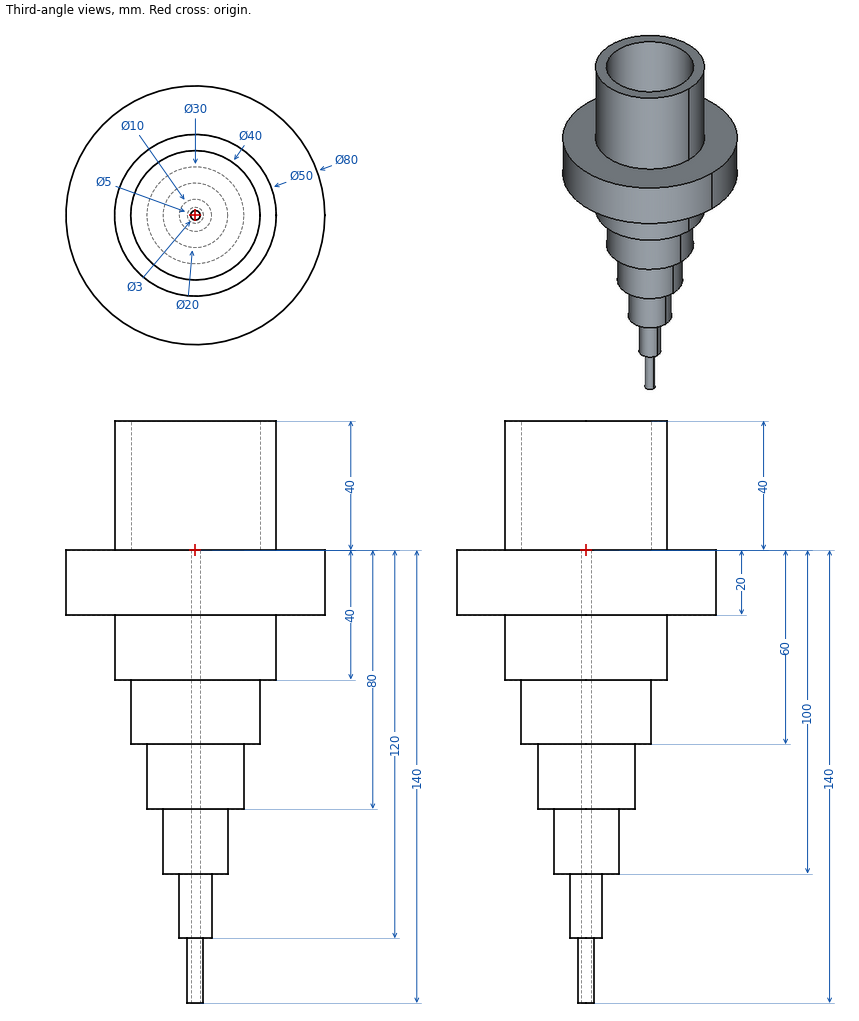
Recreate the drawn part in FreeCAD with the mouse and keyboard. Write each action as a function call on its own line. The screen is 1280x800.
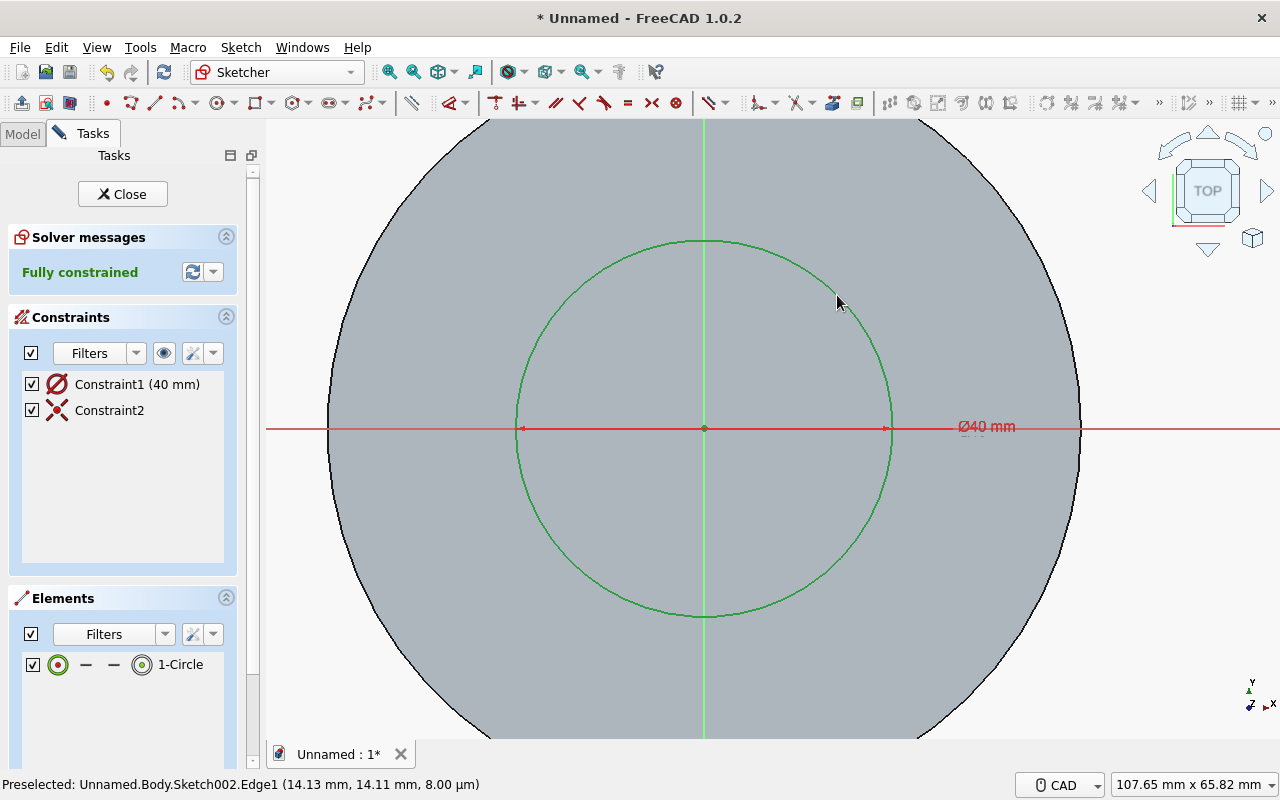
click(123, 194)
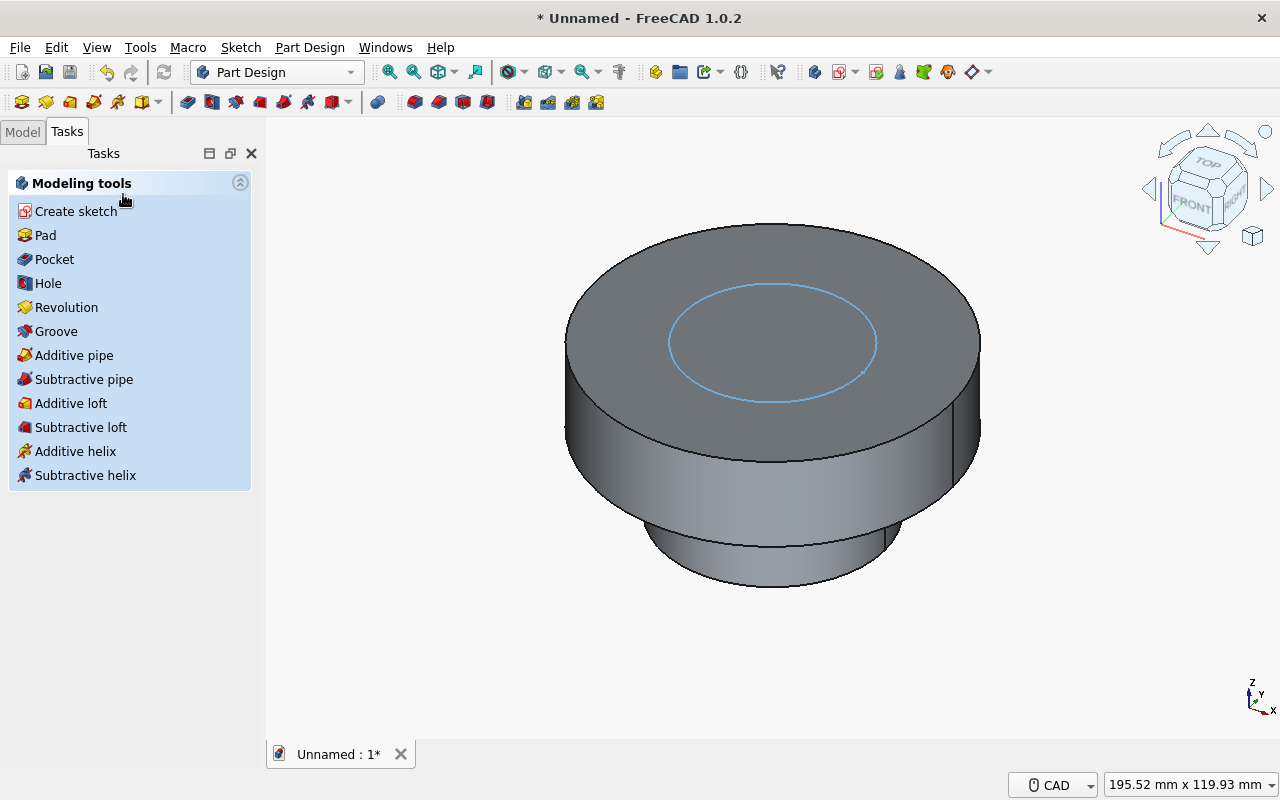
click(22, 102)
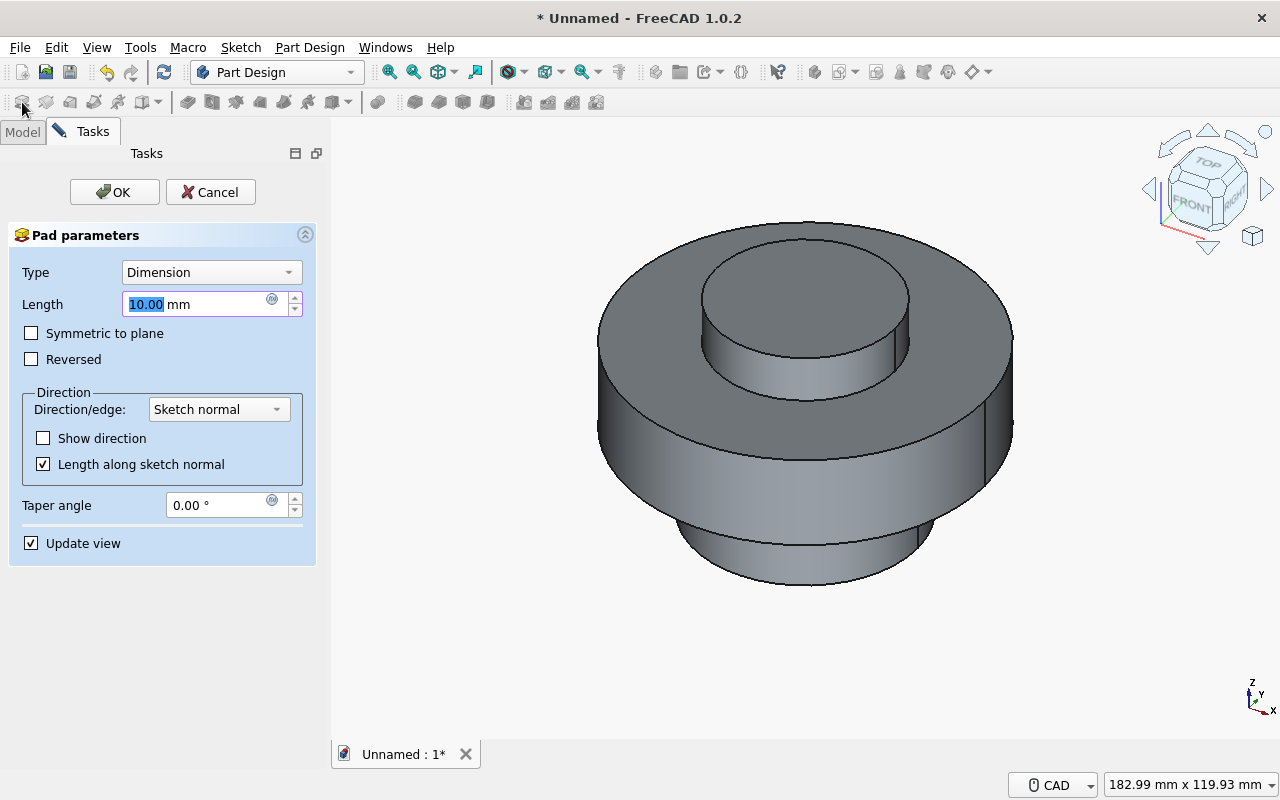
text(60)
key(Tab)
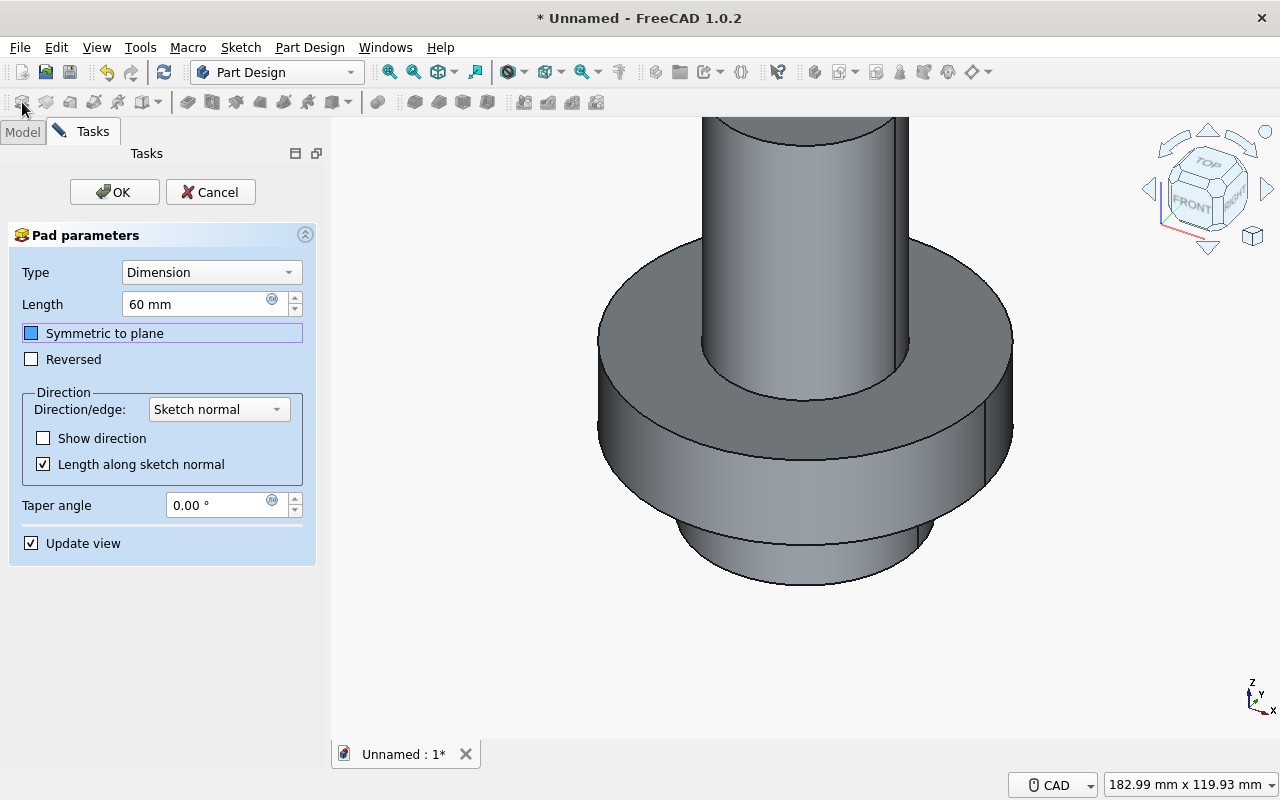
click(30, 359)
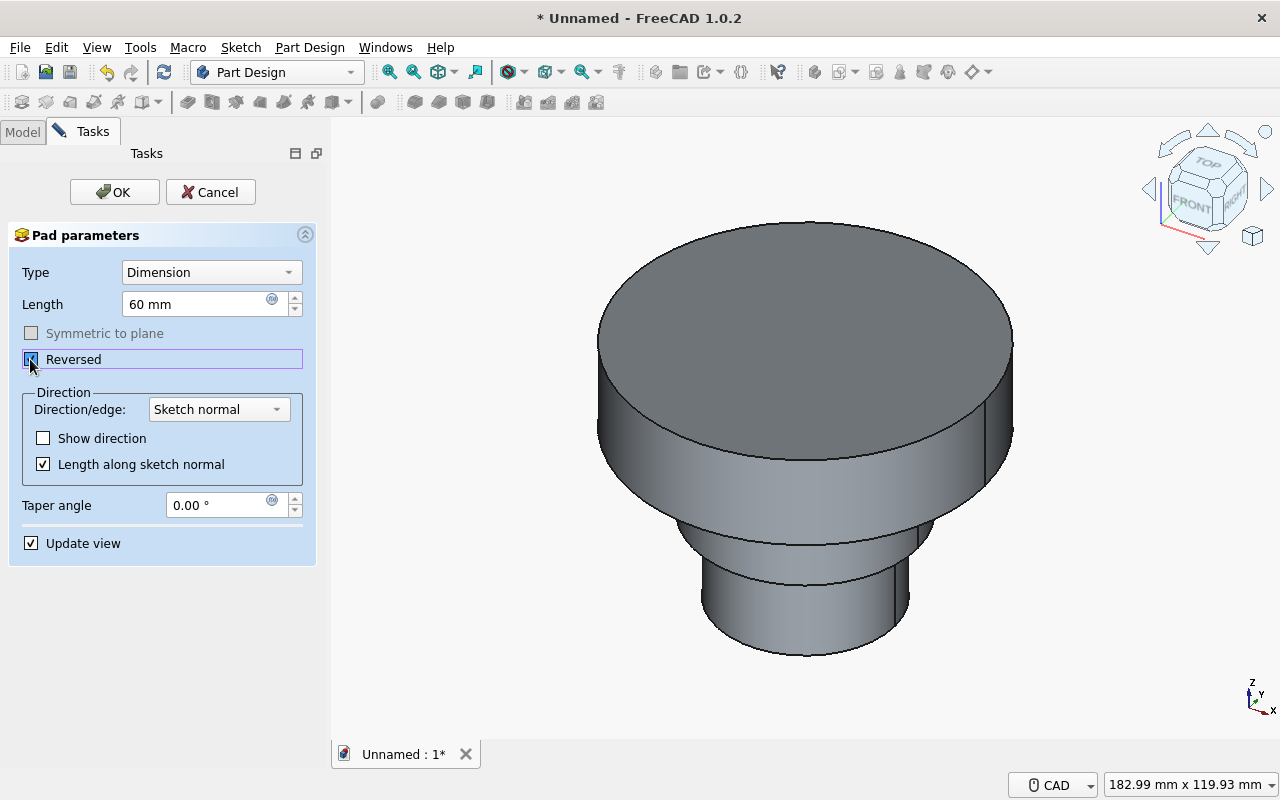
click(115, 192)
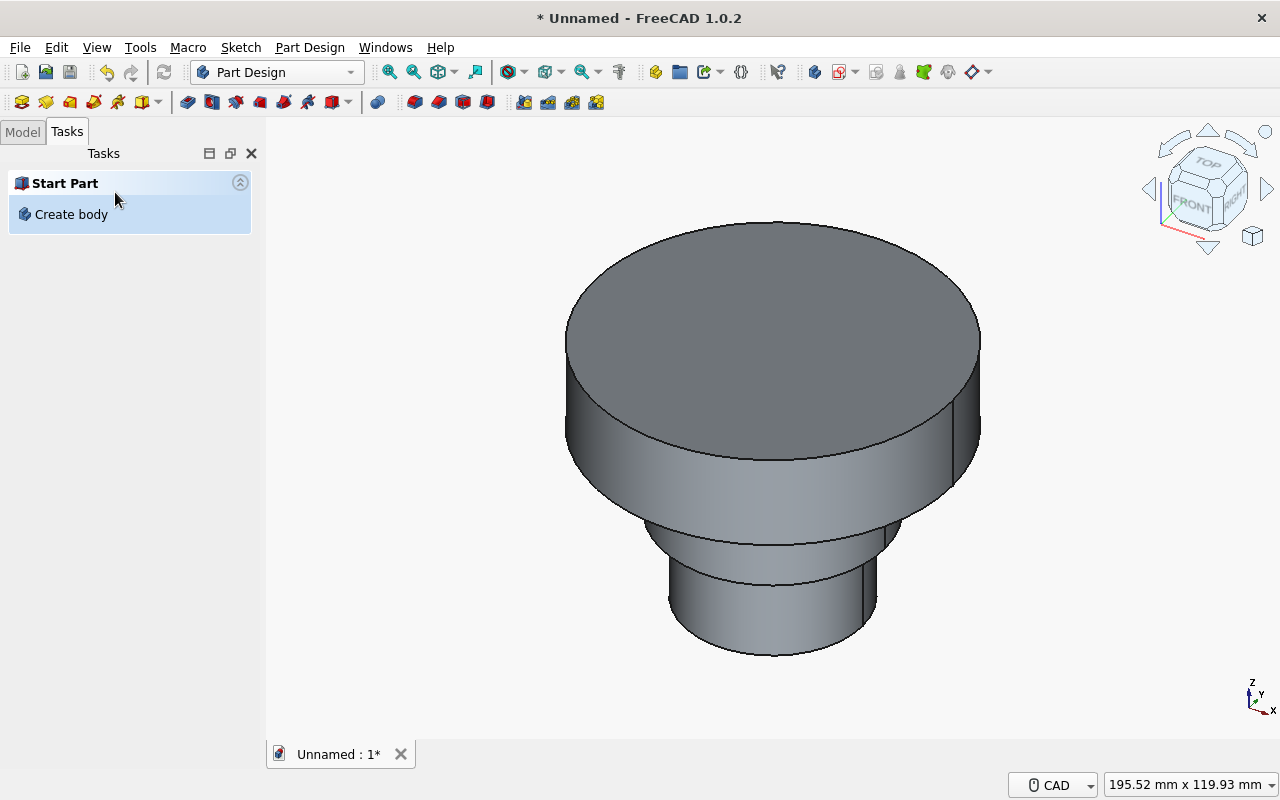
key(v)
key(f)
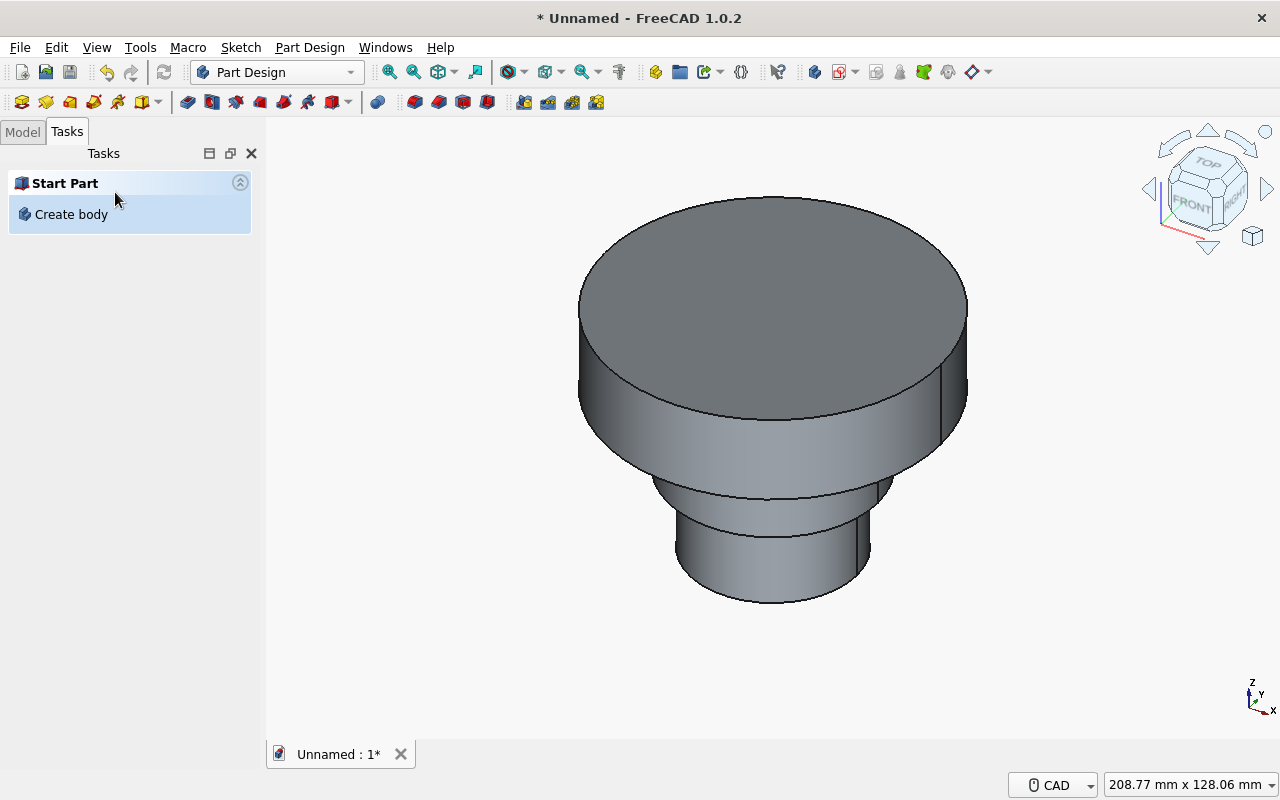
click(773, 308)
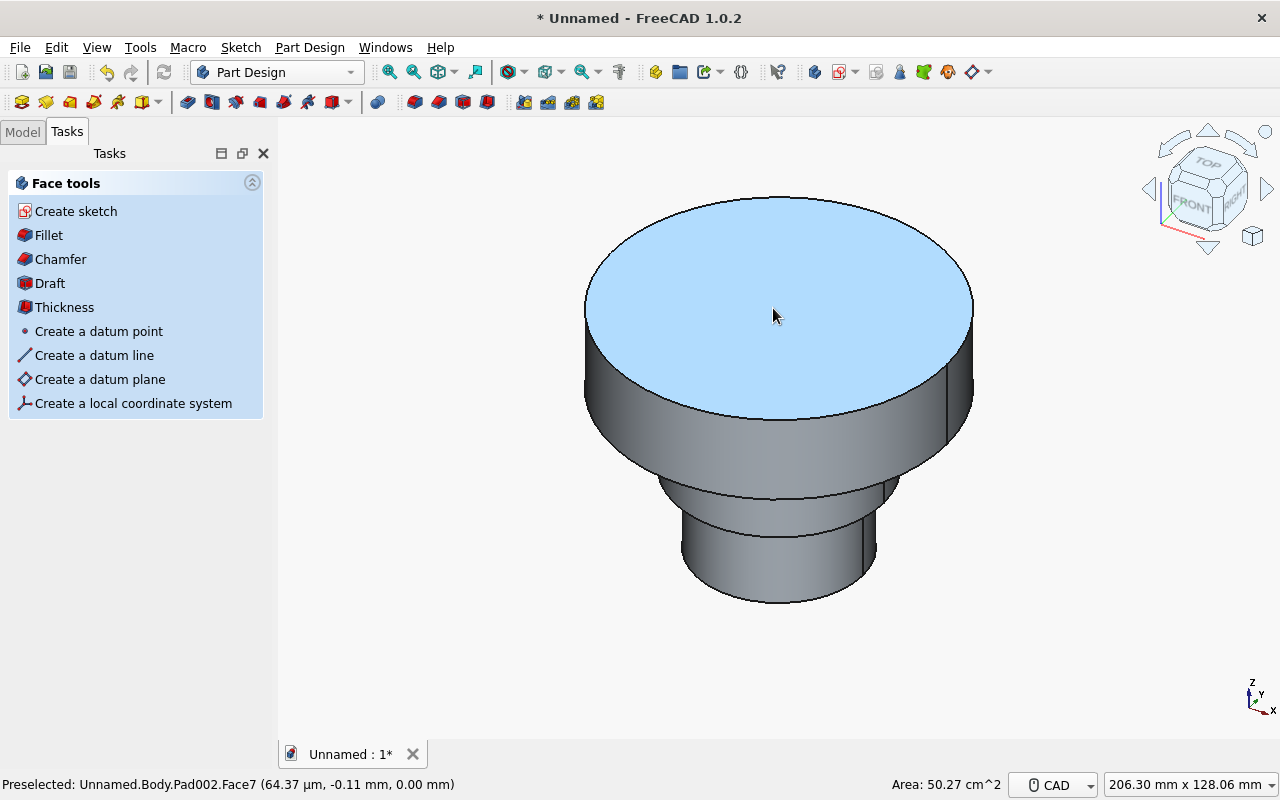
click(840, 72)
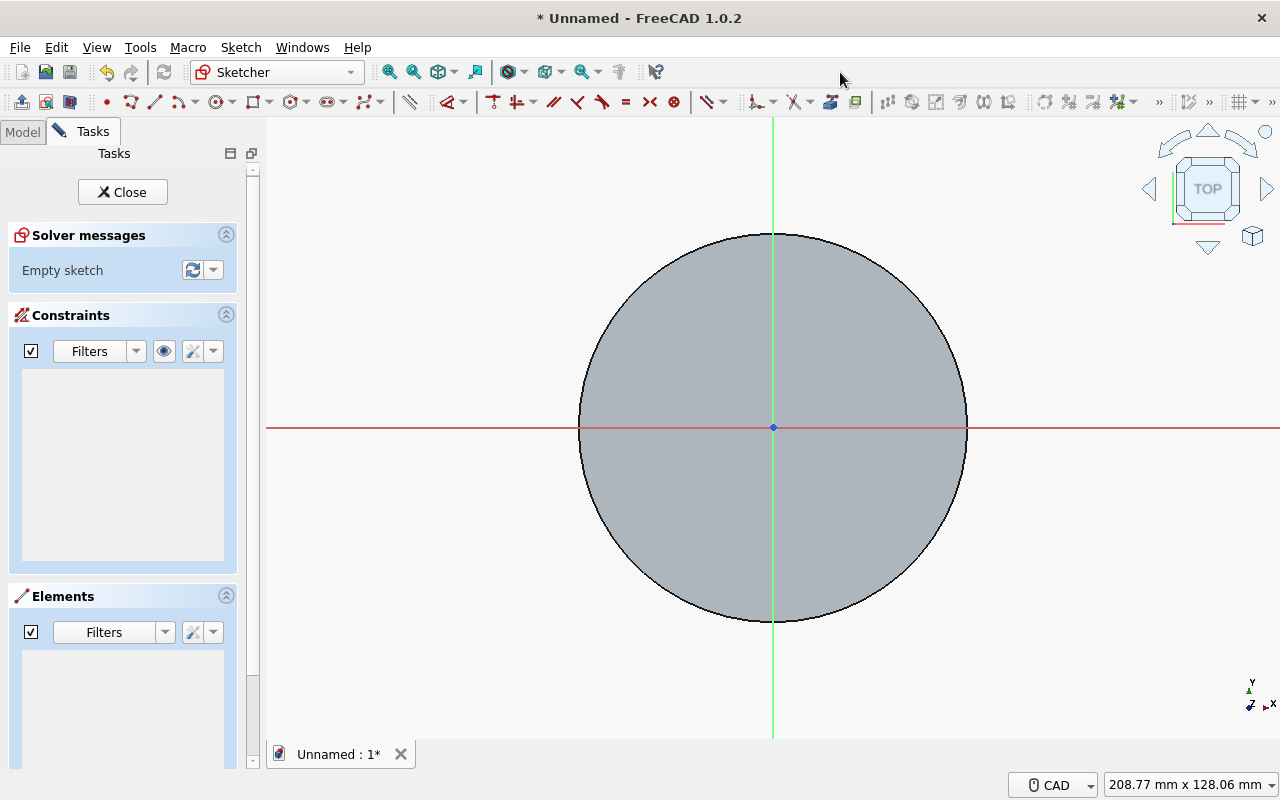
scroll(813, 428, up, 5)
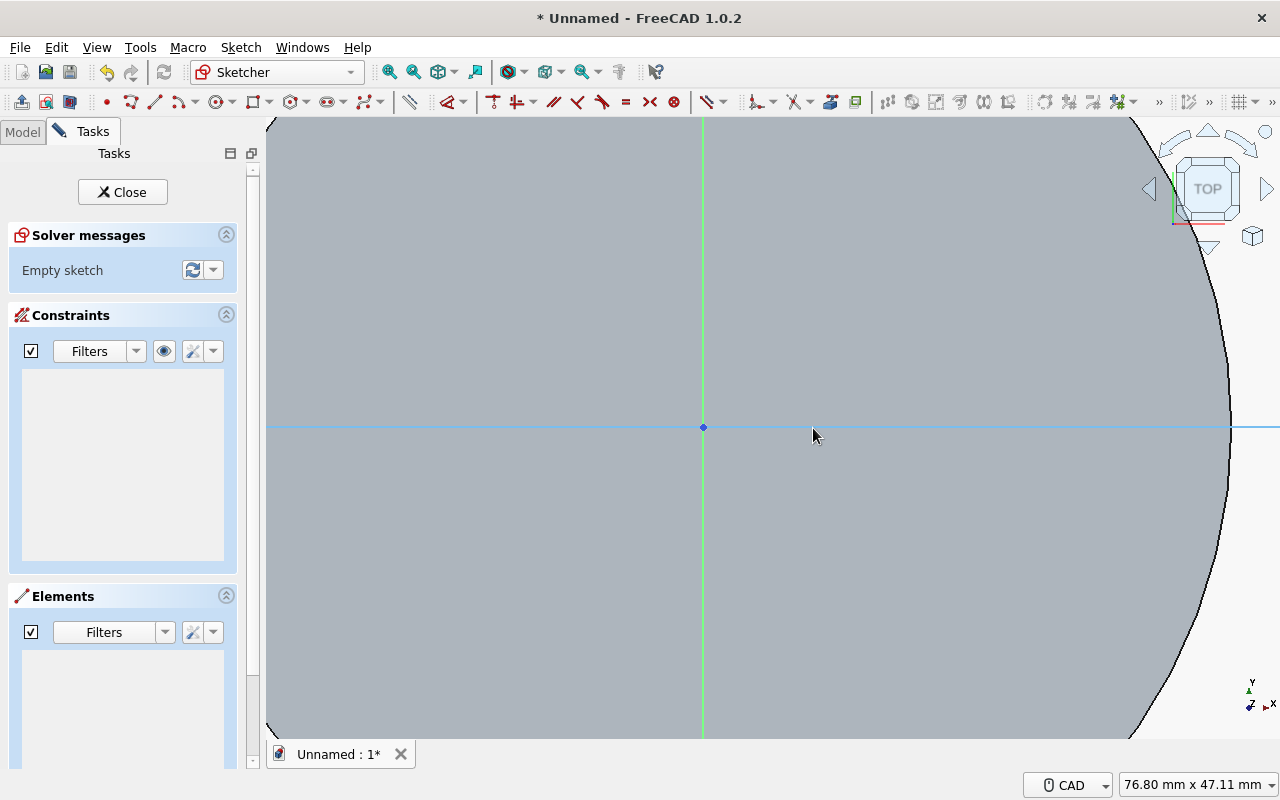
key(g)
key(c)